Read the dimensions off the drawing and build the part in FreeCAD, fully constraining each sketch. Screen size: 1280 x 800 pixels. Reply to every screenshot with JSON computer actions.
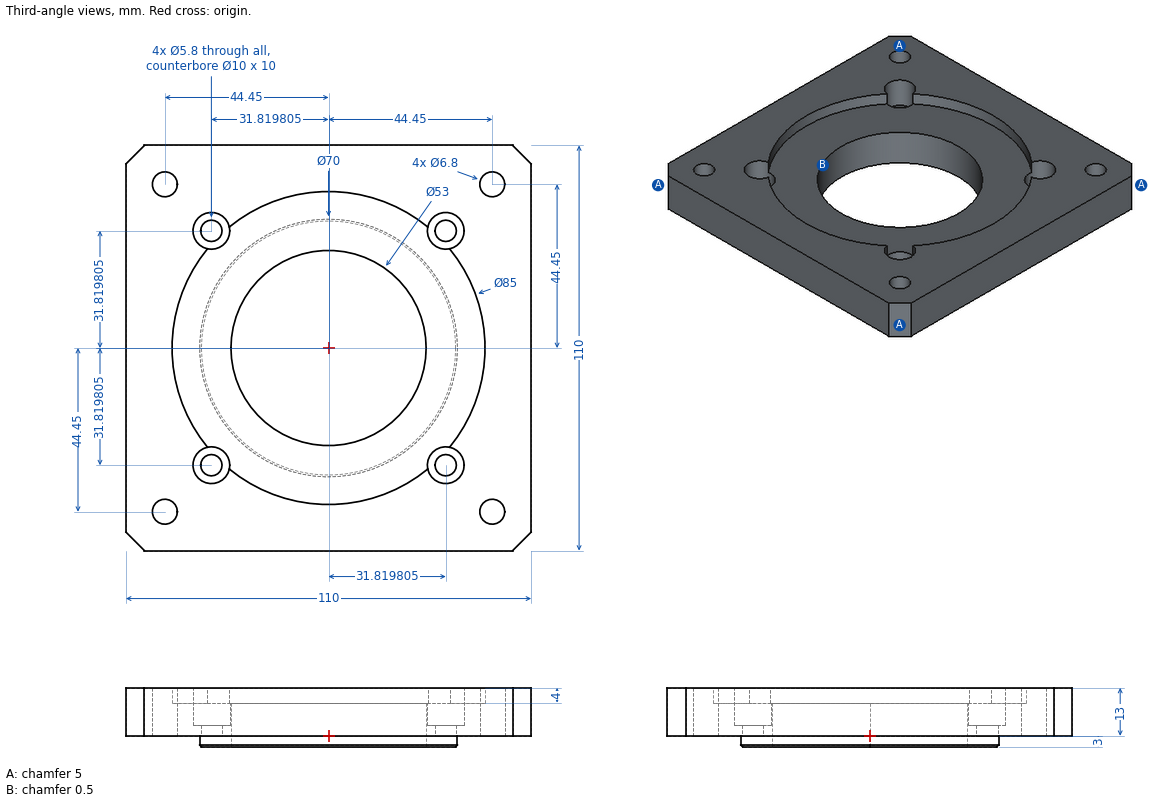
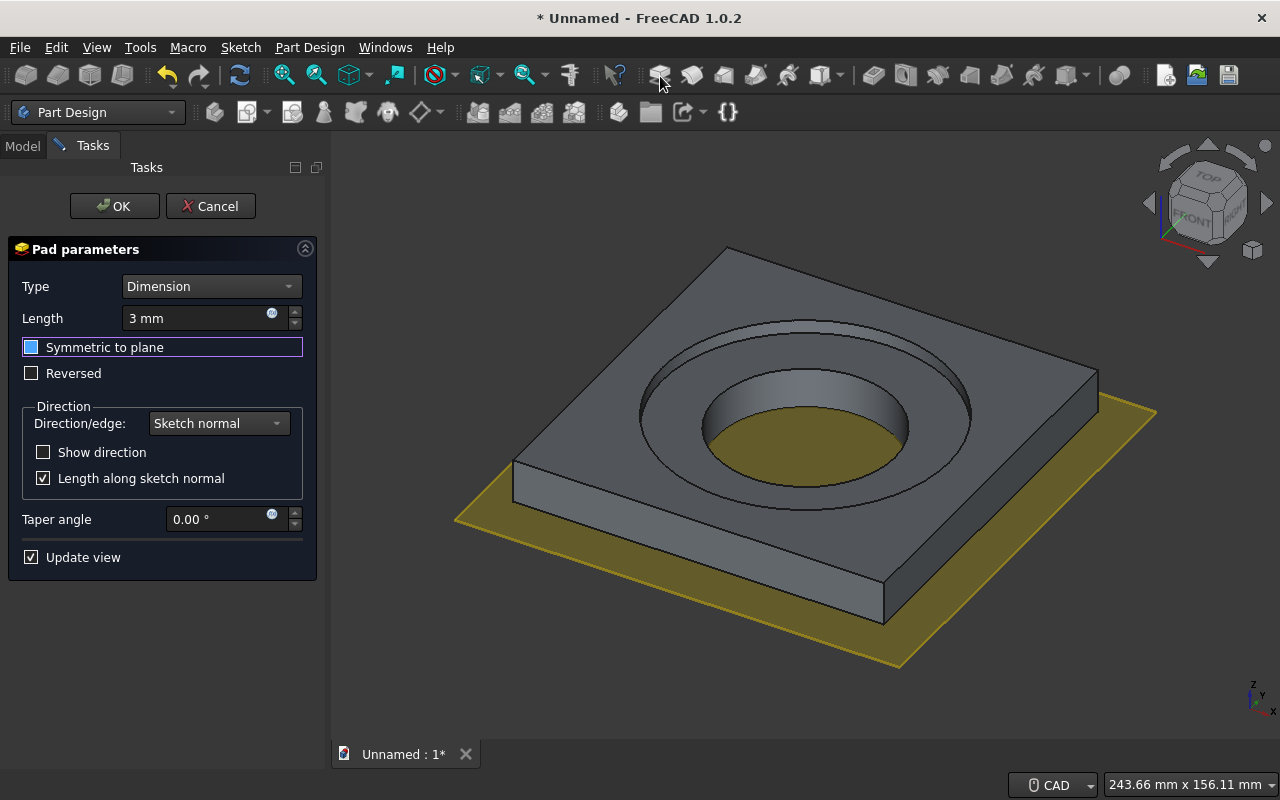
{"action": "left_click", "coordinate": [115, 206]}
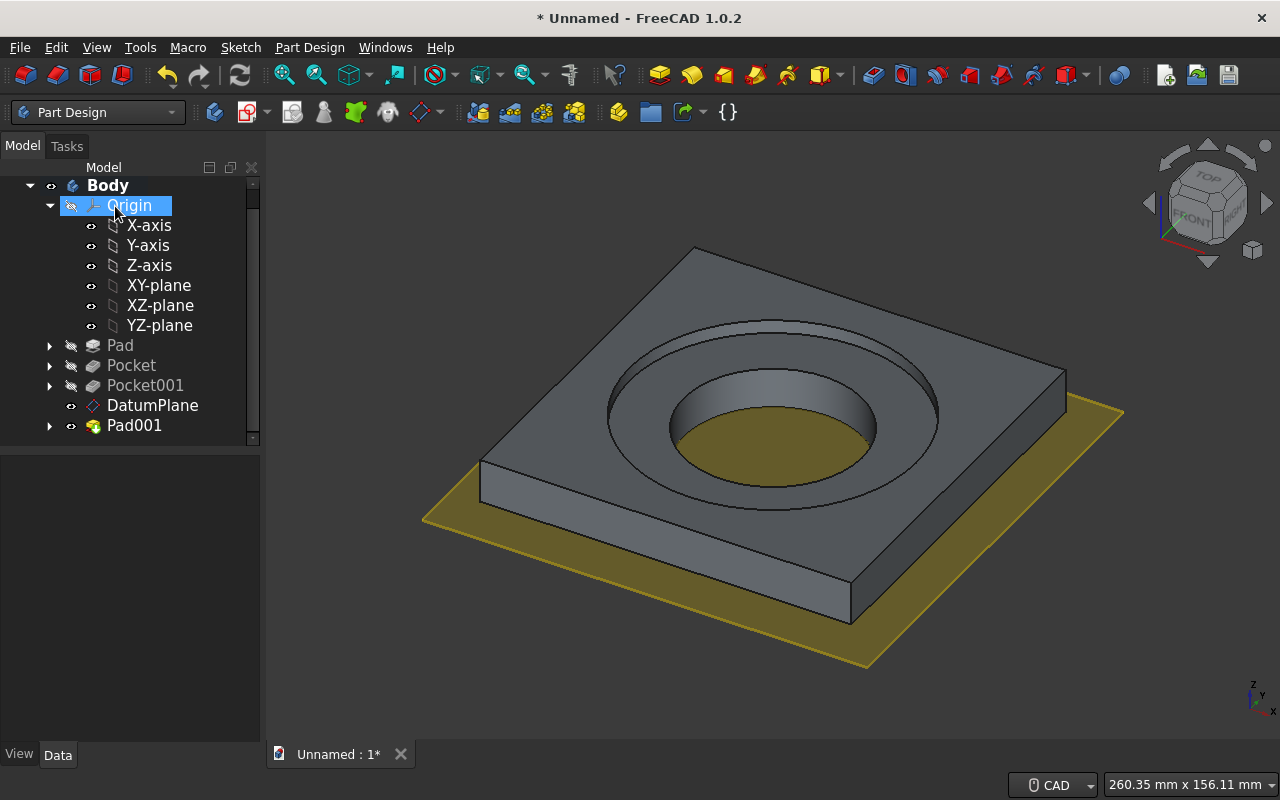
{"action": "left_click", "coordinate": [116, 406]}
{"action": "key", "text": "space"}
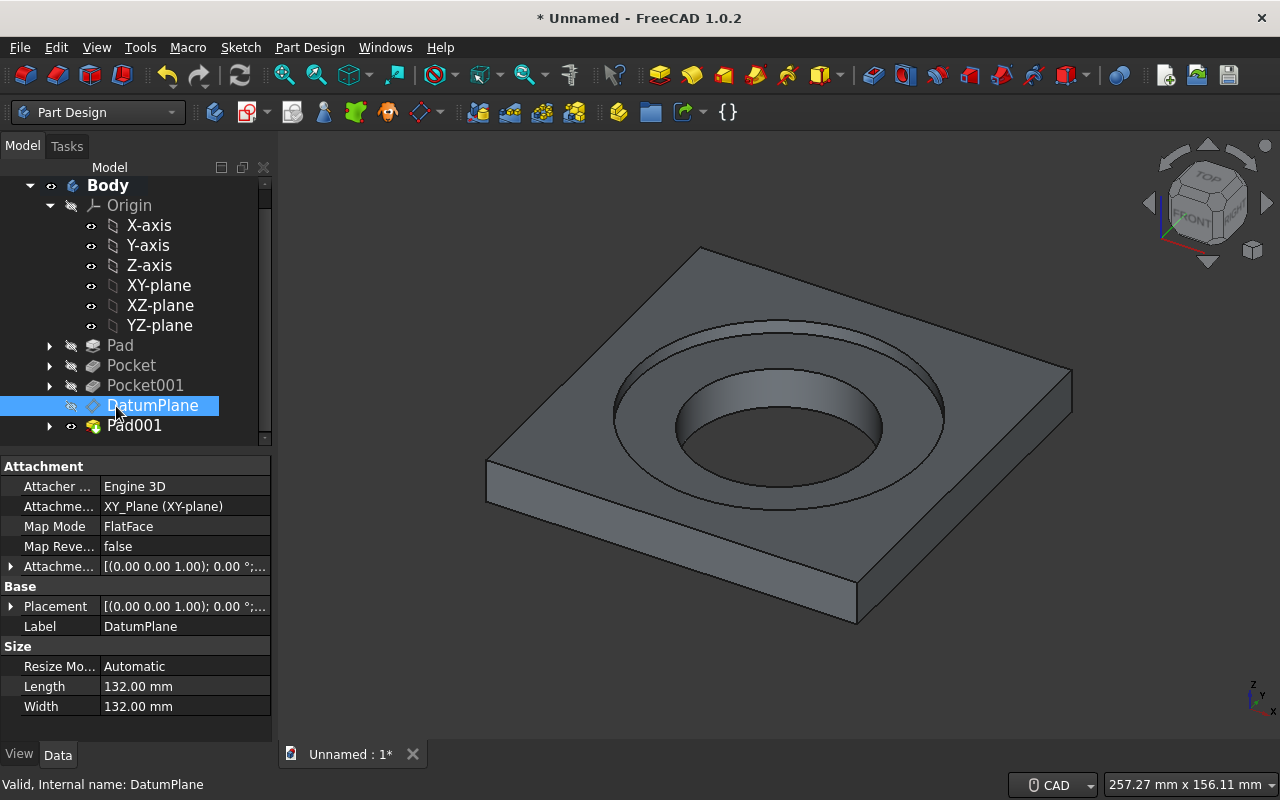
{"action": "key", "text": "5"}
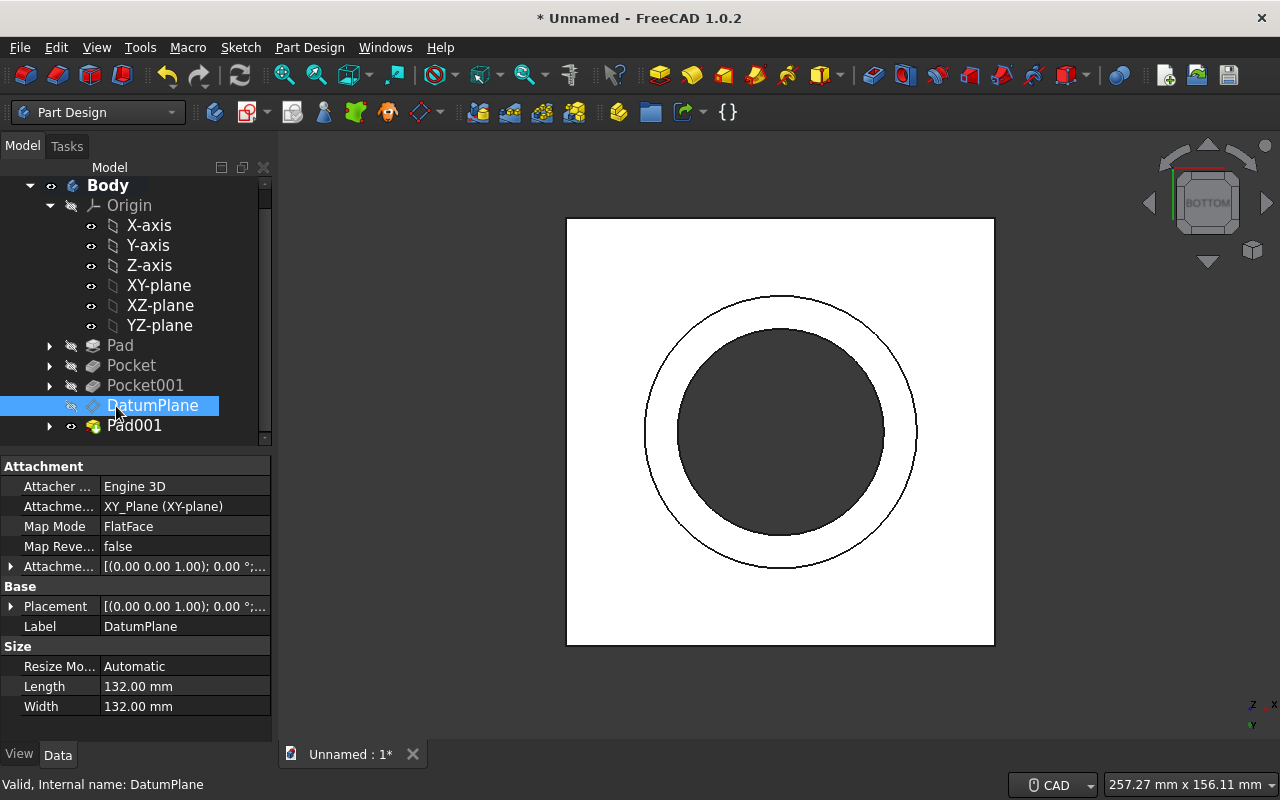
{"action": "left_click", "coordinate": [903, 554]}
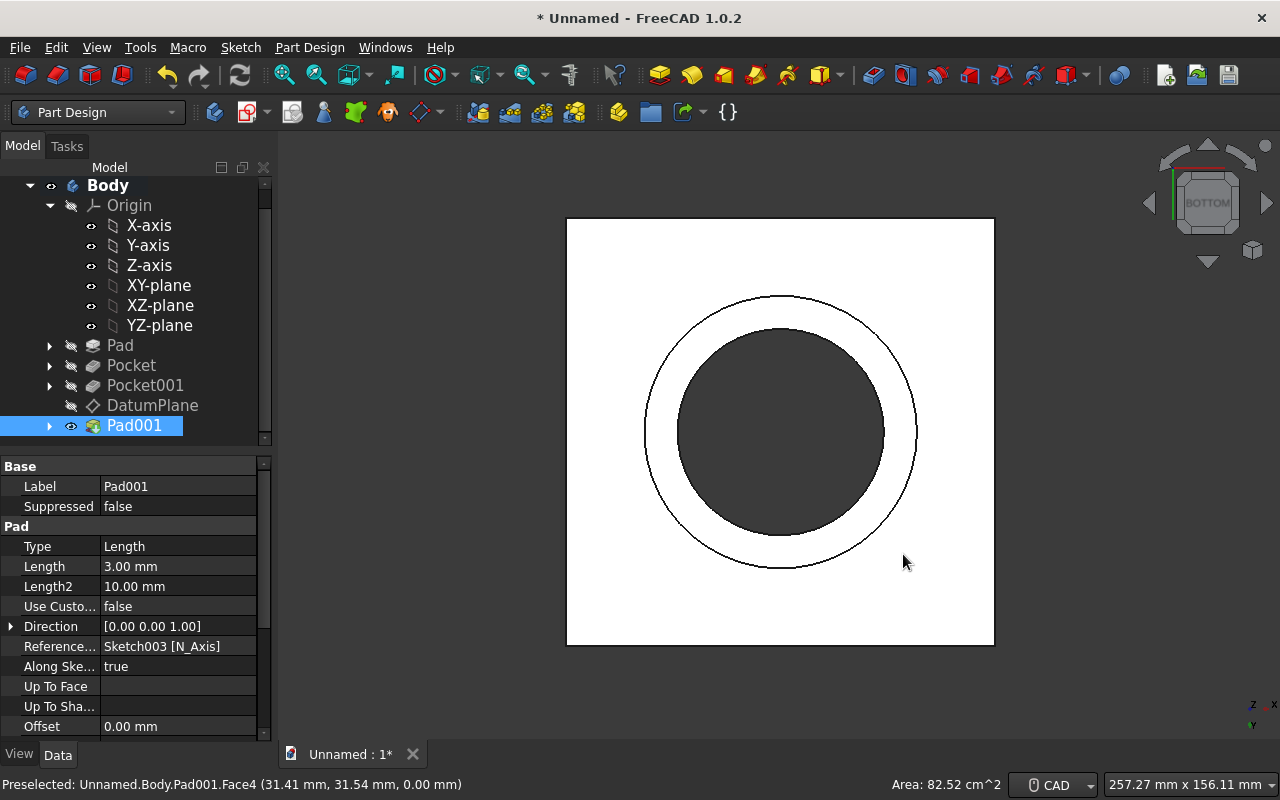
{"action": "left_click", "coordinate": [248, 112]}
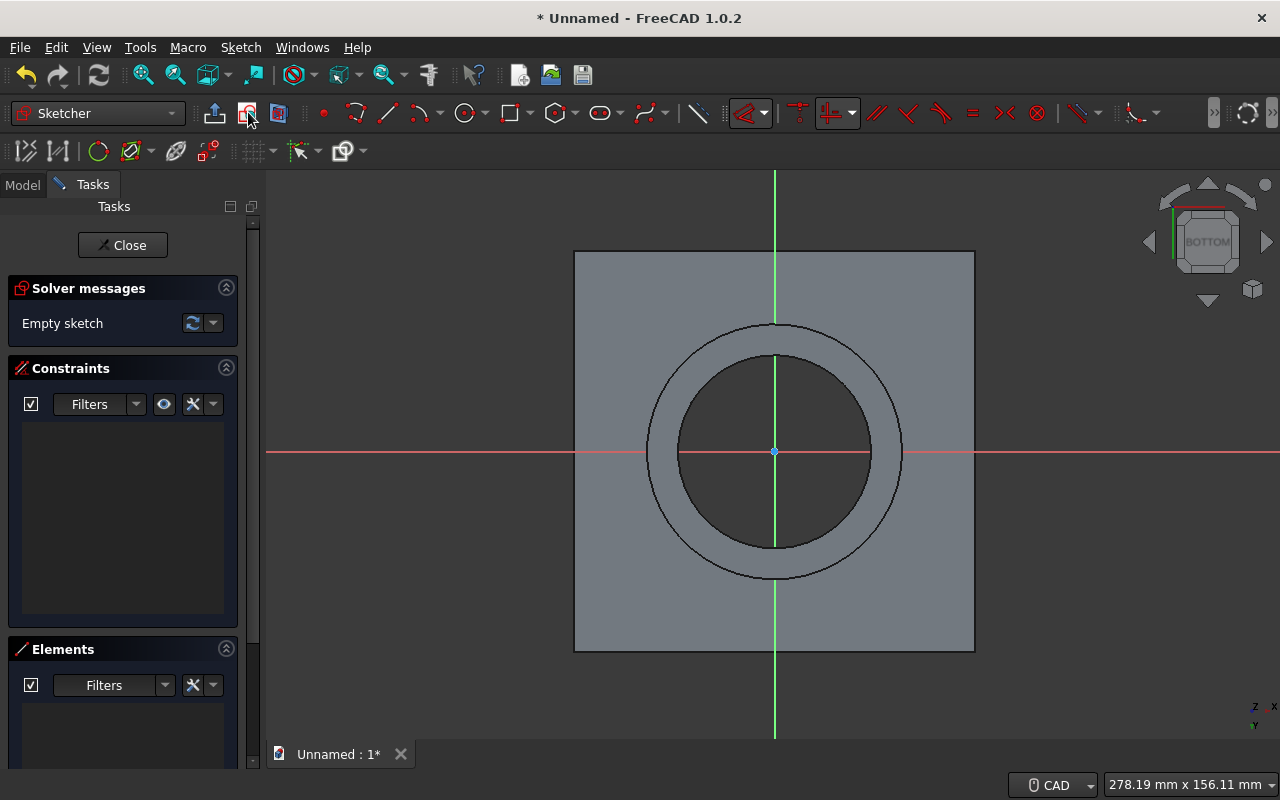
{"action": "left_click", "coordinate": [280, 114]}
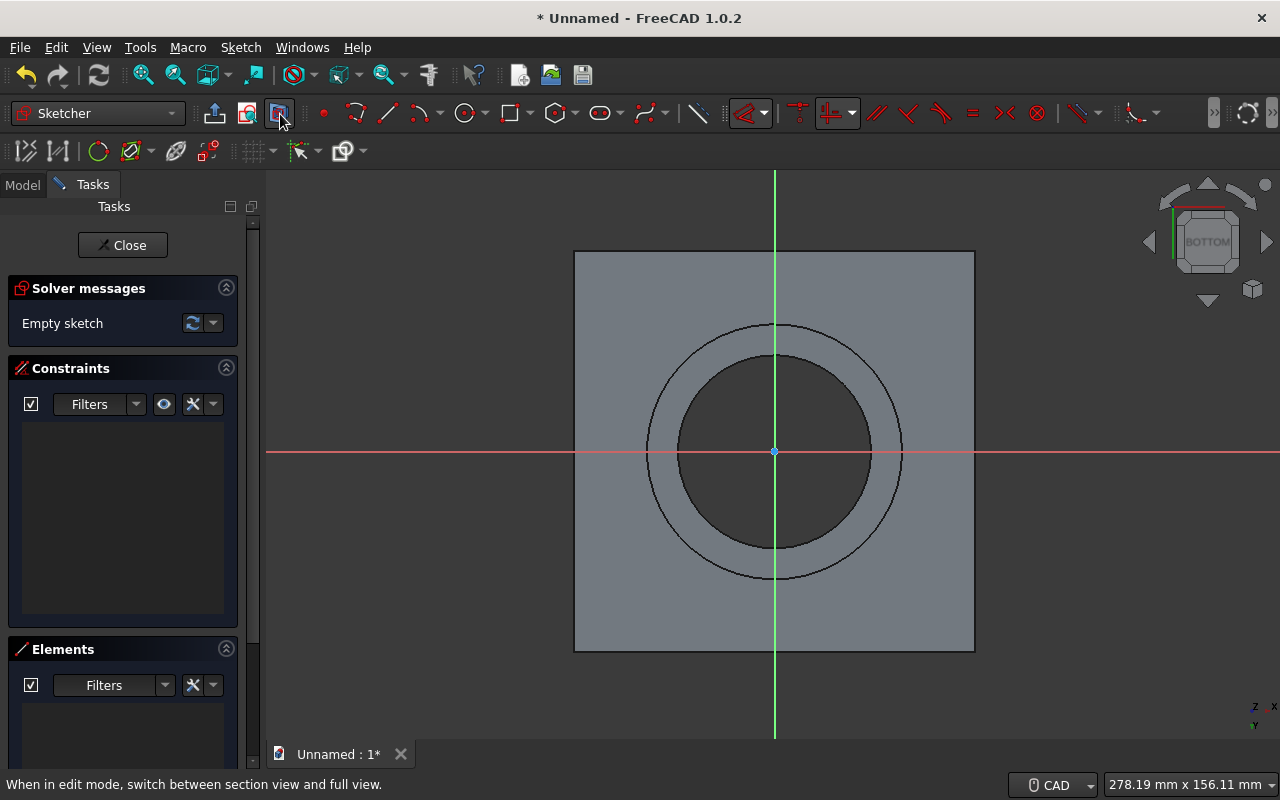
{"action": "left_click", "coordinate": [466, 114]}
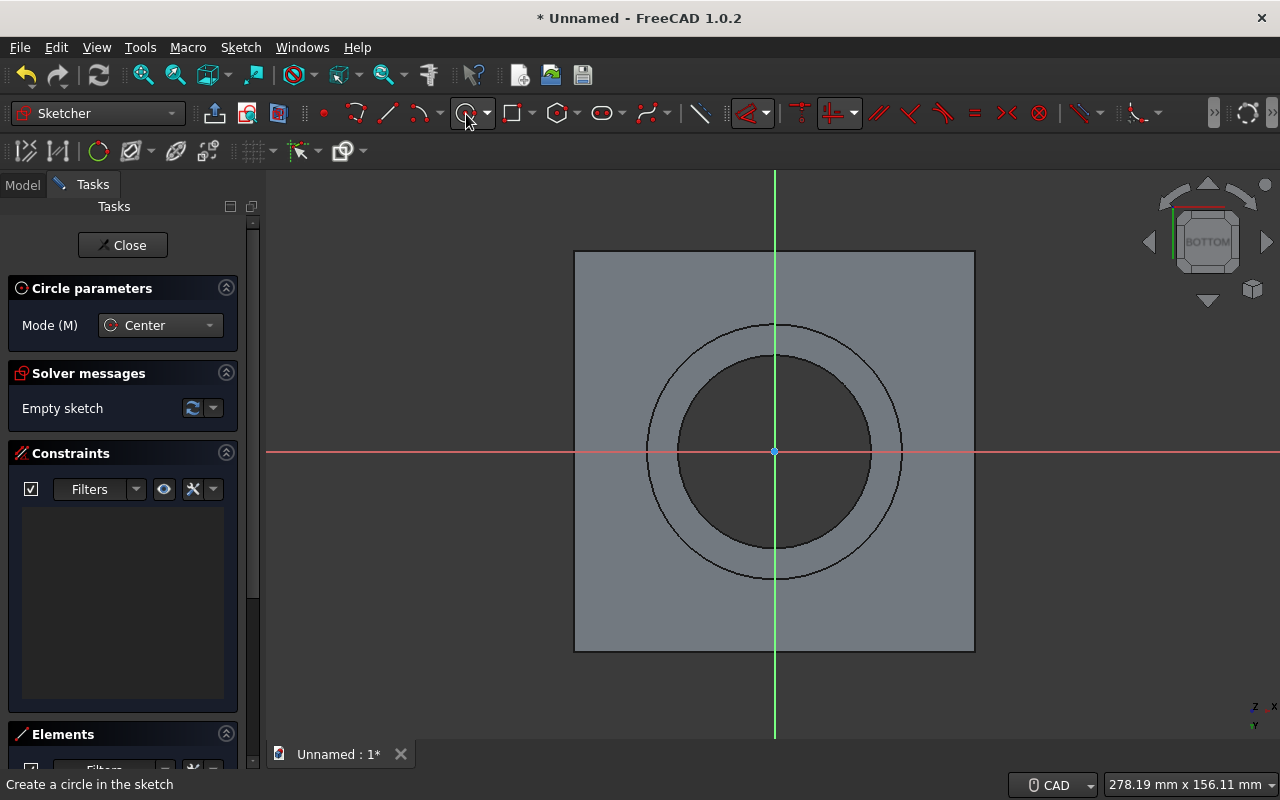
{"action": "scroll", "coordinate": [937, 614], "scroll_direction": "up", "scroll_amount": 4}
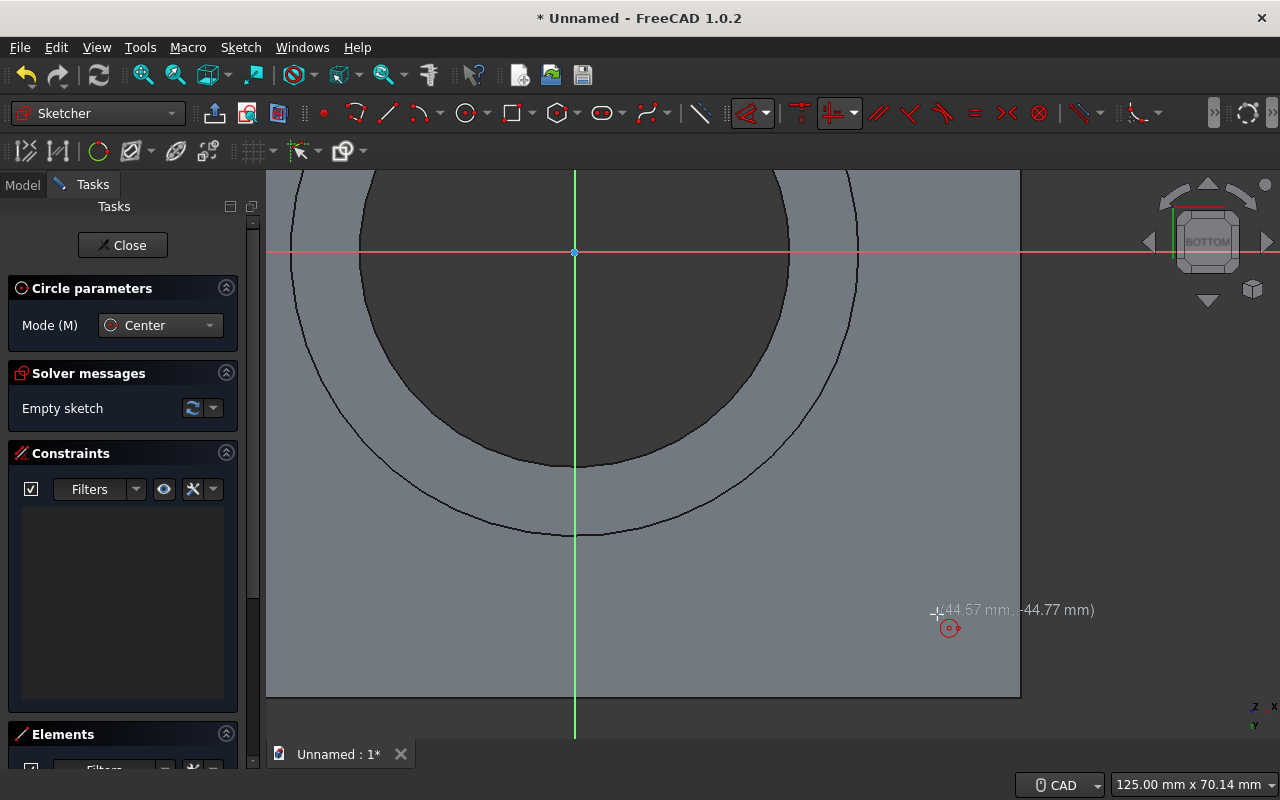
{"action": "left_click", "coordinate": [935, 613]}
{"action": "left_click", "coordinate": [955, 593]}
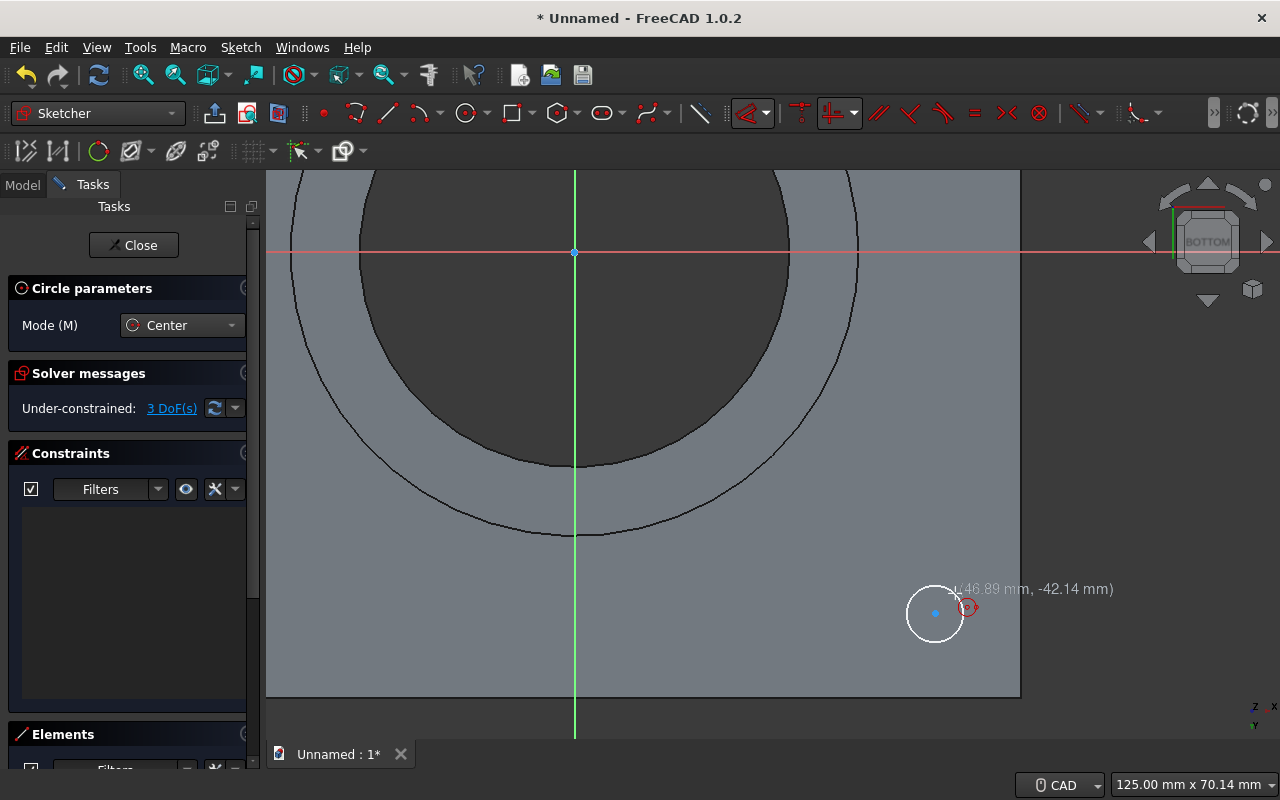
{"action": "scroll", "coordinate": [810, 620], "scroll_direction": "down", "scroll_amount": 4}